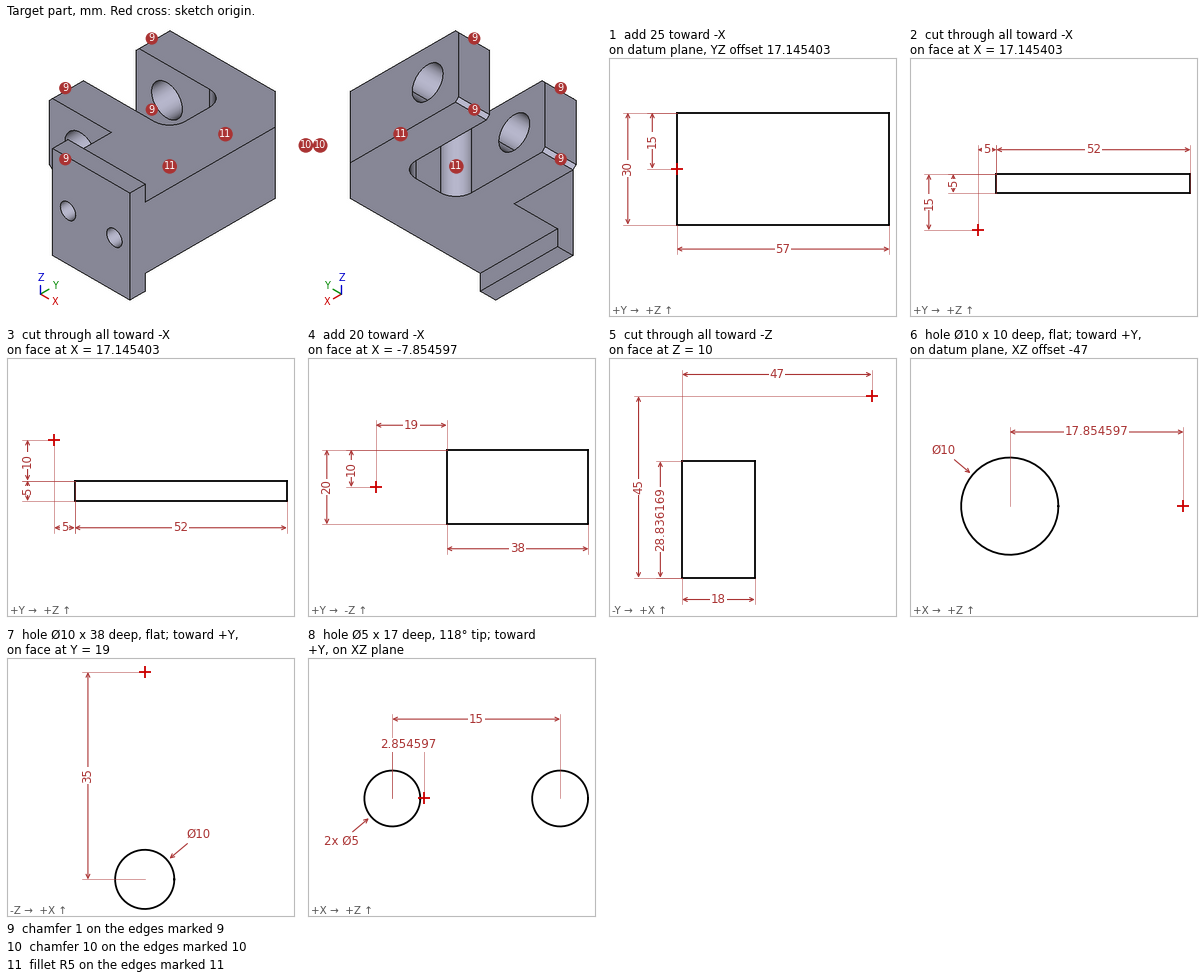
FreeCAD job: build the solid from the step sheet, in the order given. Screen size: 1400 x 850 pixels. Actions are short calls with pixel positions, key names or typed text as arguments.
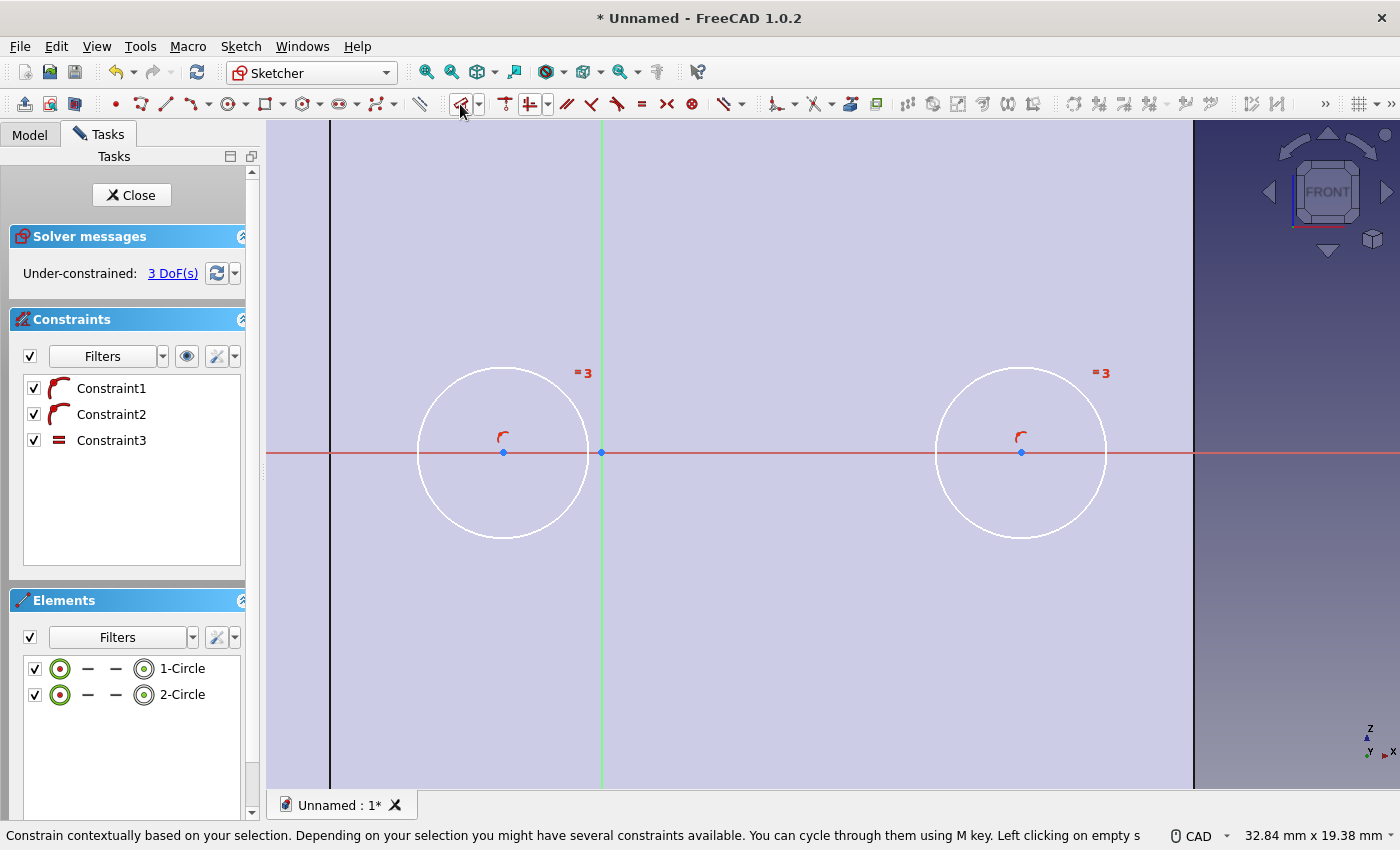
click(563, 392)
click(585, 369)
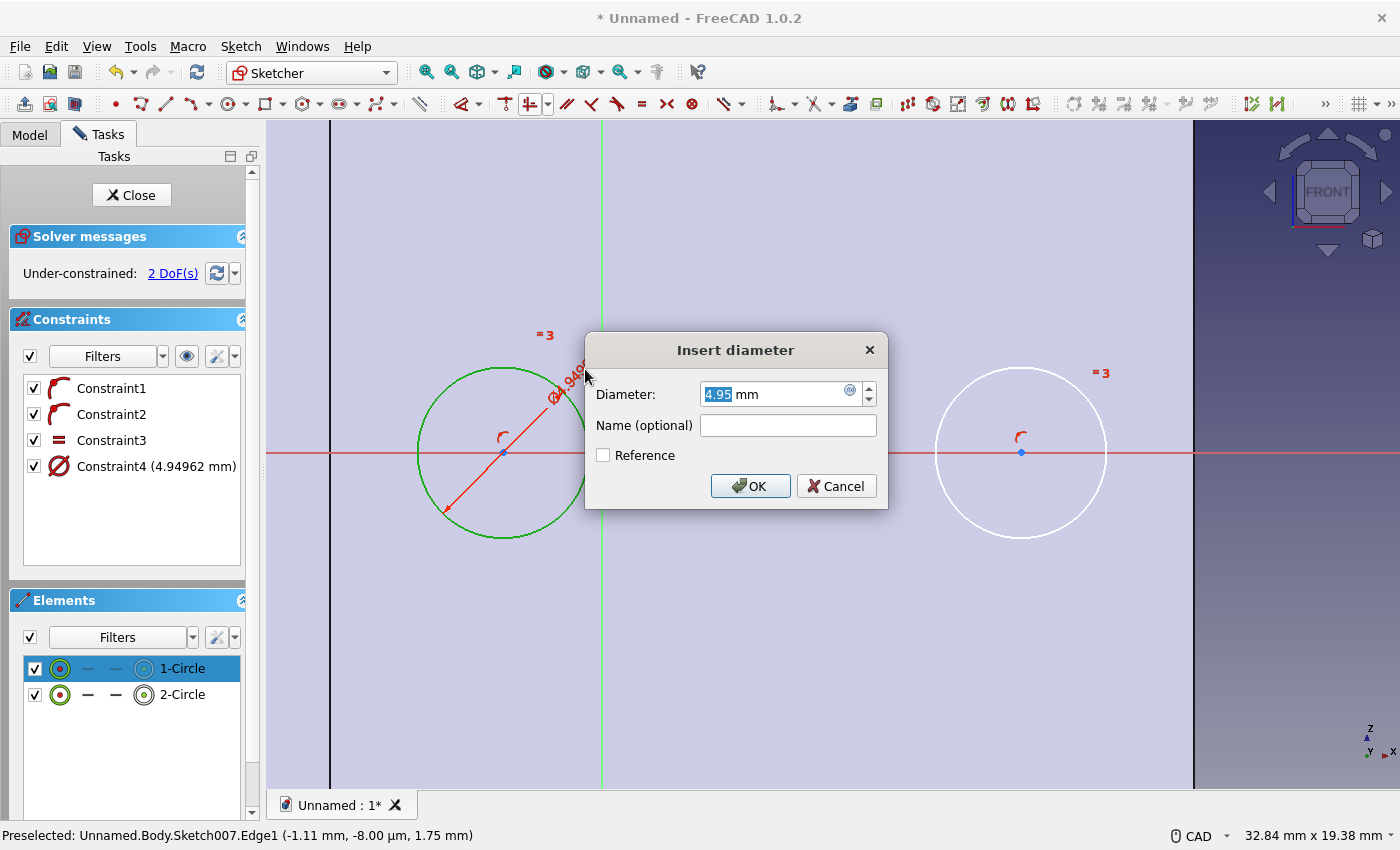
text(5)
key(Return)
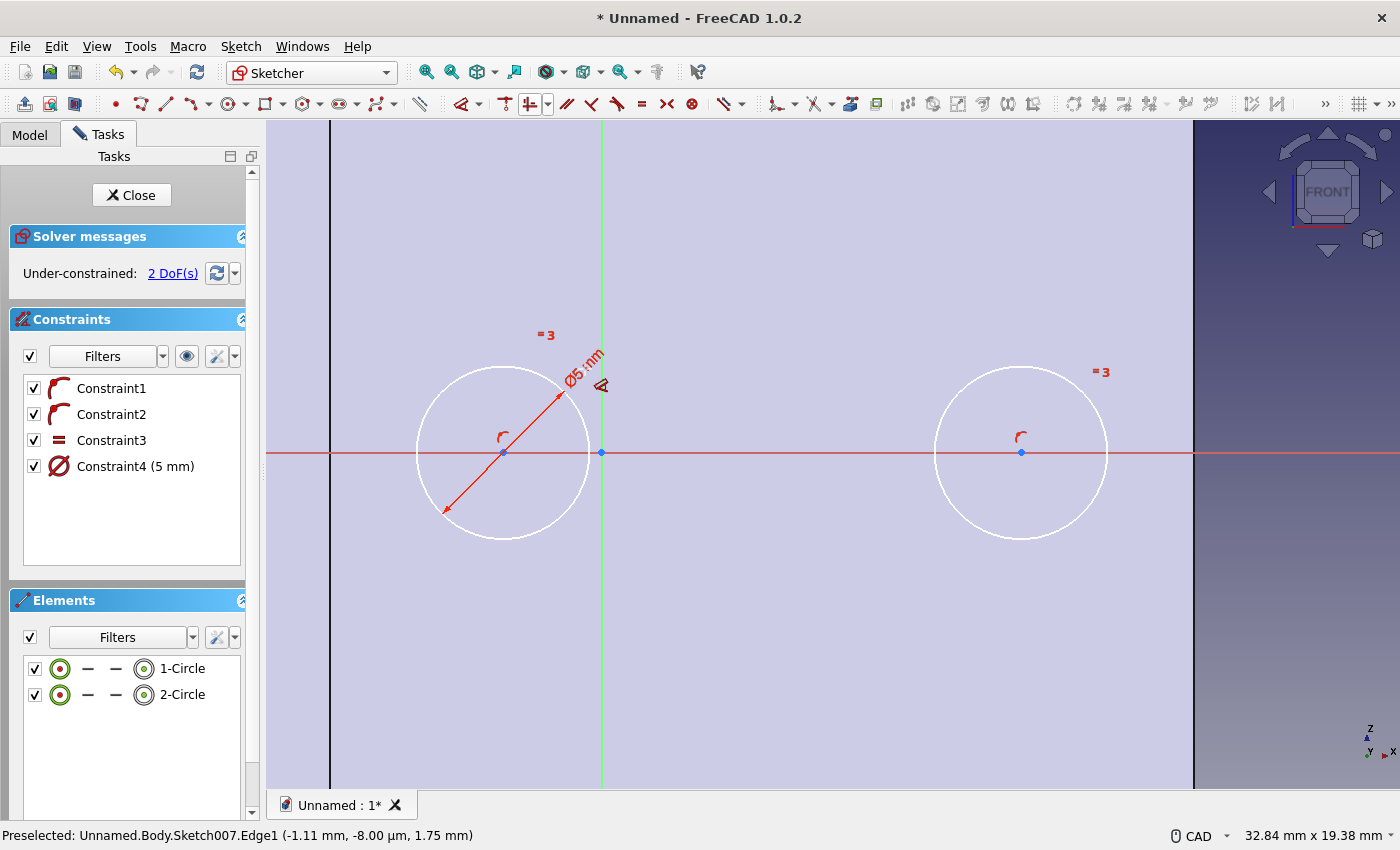
click(503, 453)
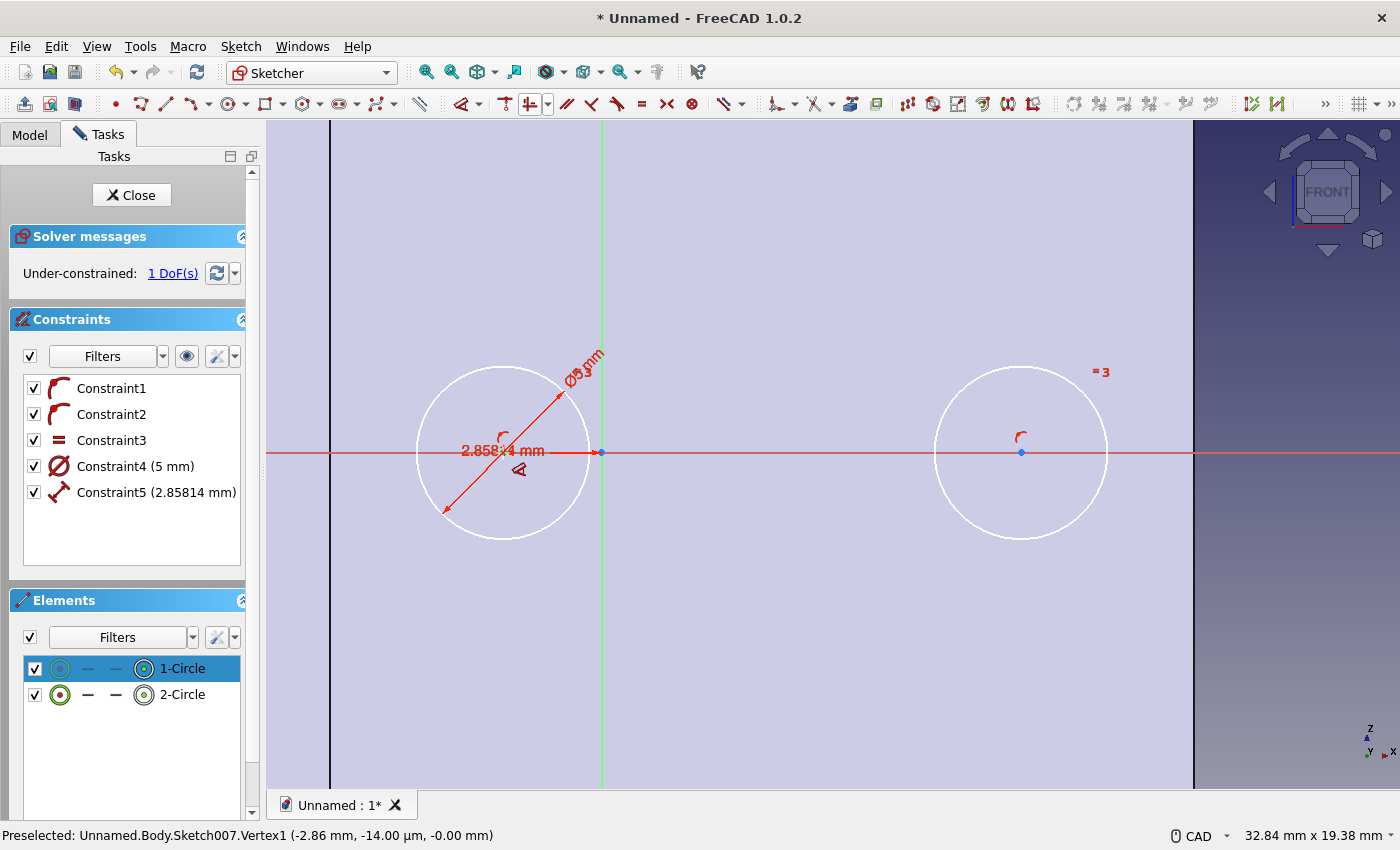
click(1021, 453)
click(762, 487)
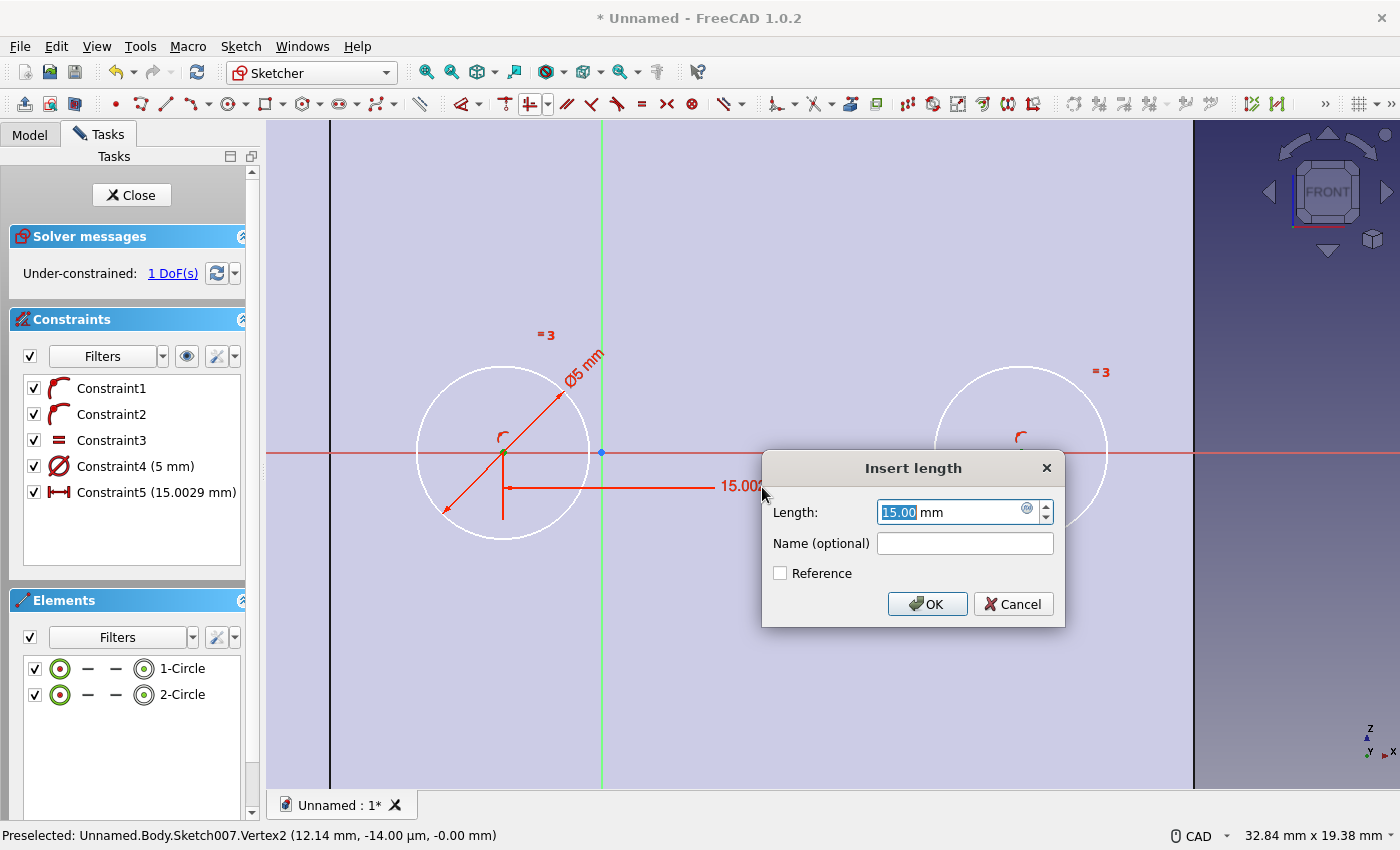
text(15)
key(Return)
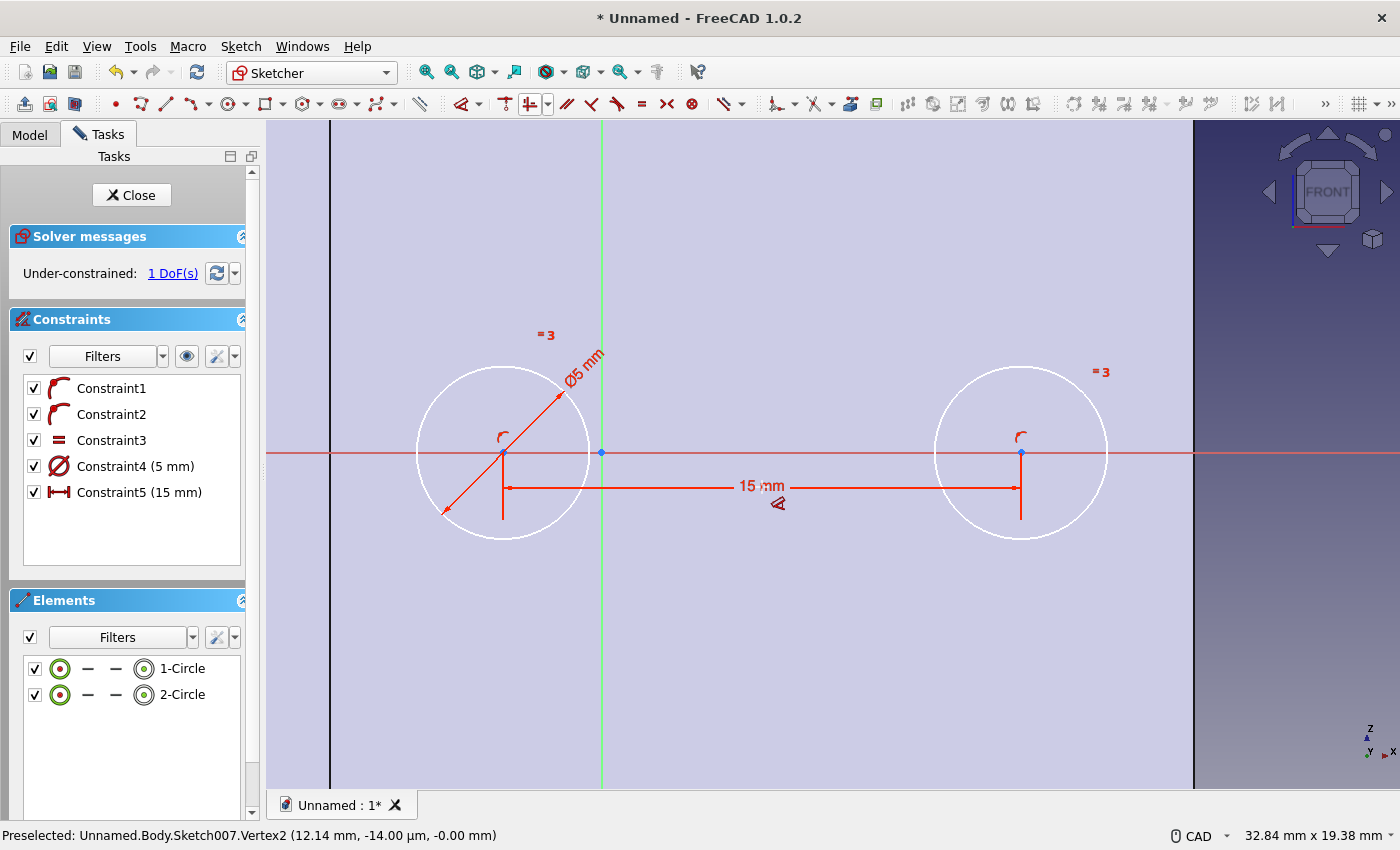
click(503, 453)
click(552, 487)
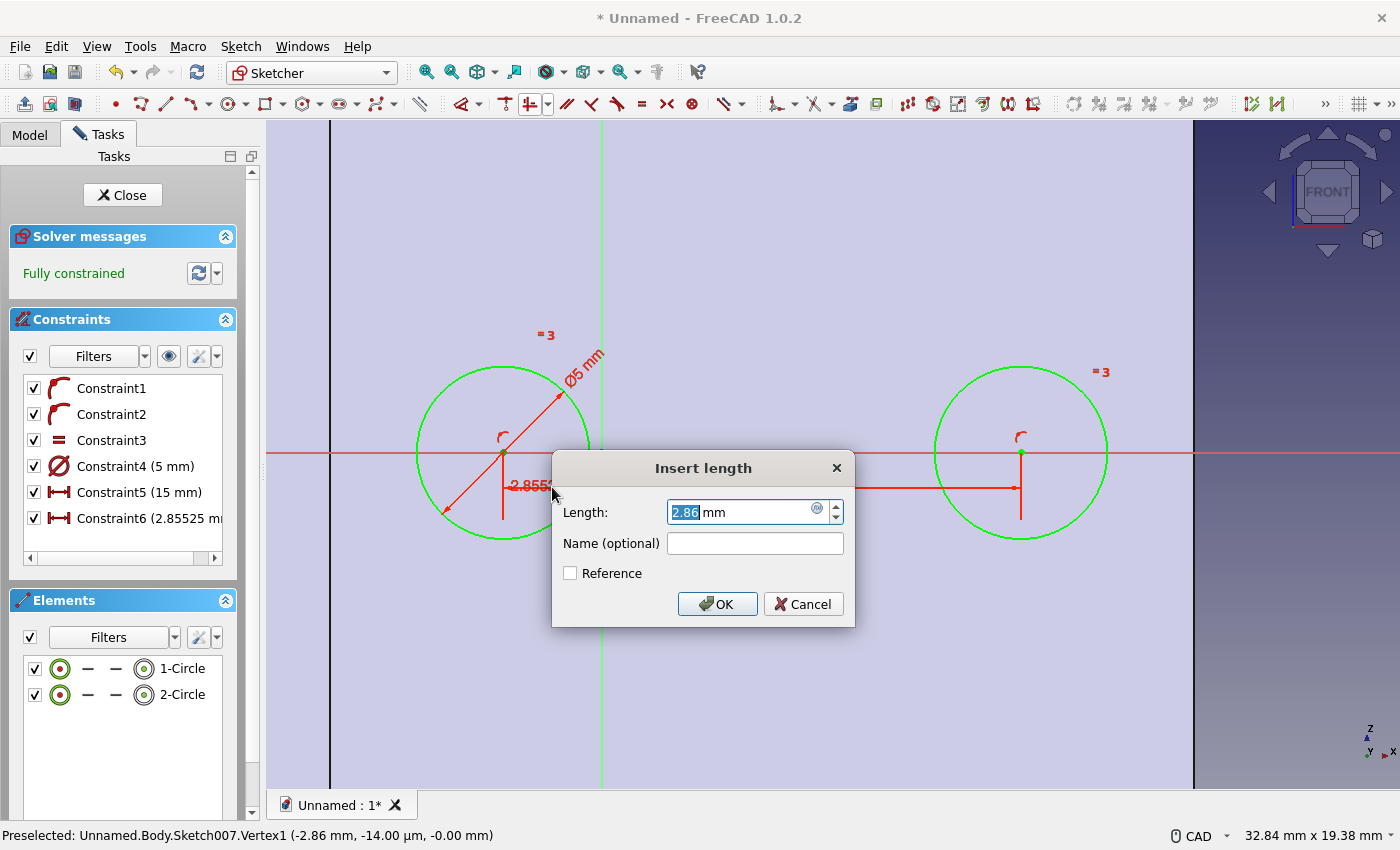
text(2.854597)
key(Return)
key(Escape)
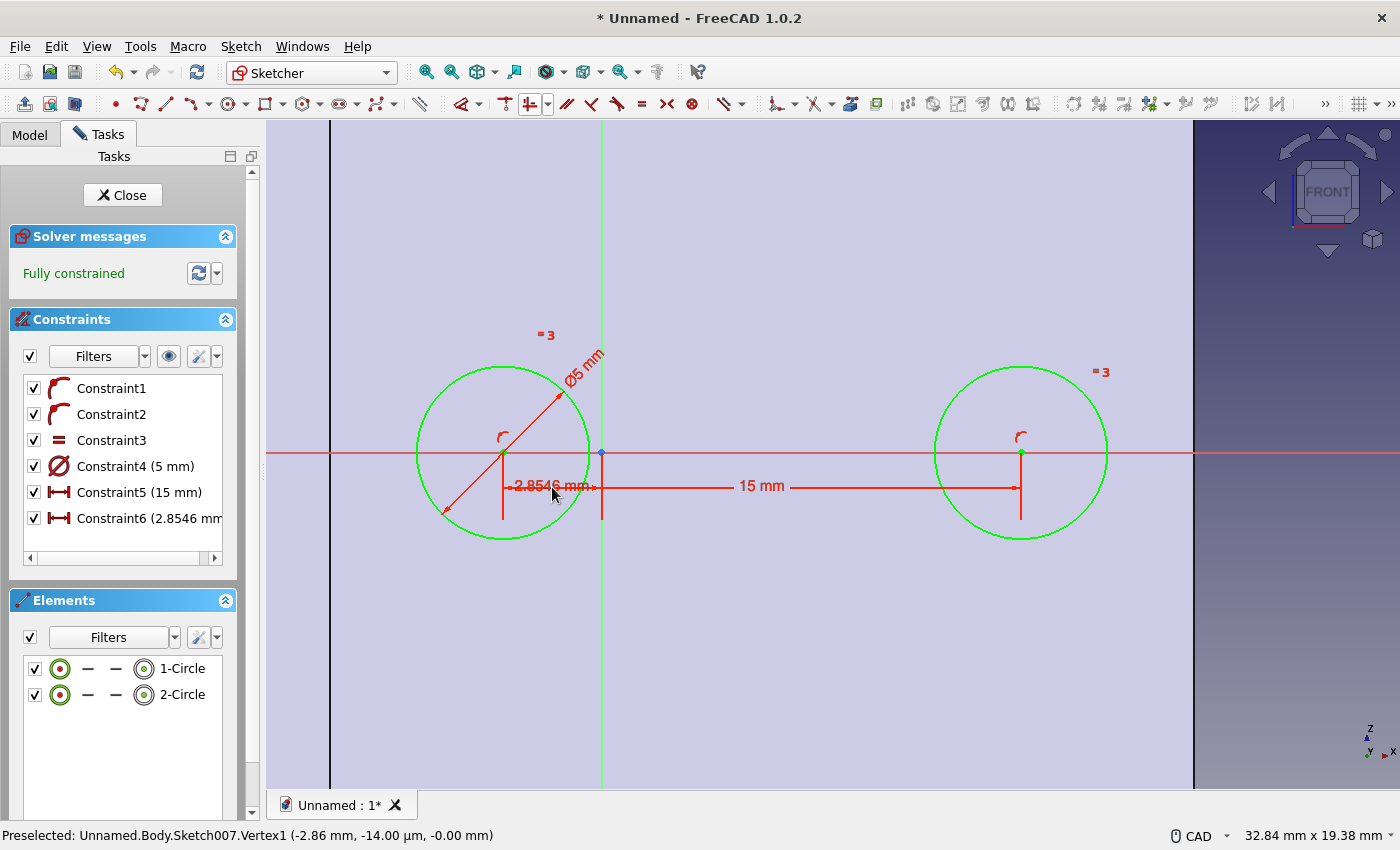
click(123, 195)